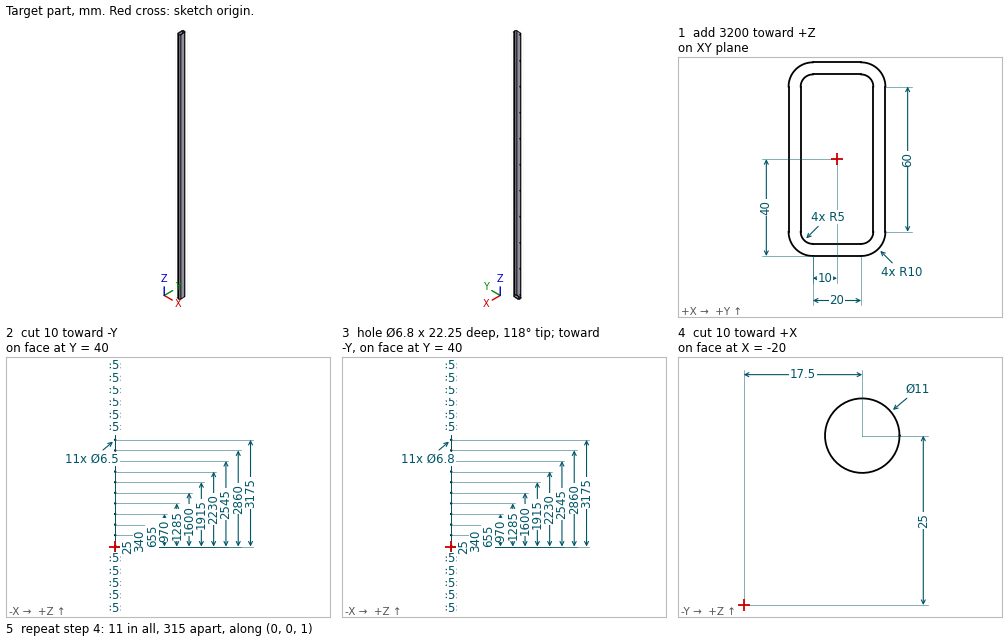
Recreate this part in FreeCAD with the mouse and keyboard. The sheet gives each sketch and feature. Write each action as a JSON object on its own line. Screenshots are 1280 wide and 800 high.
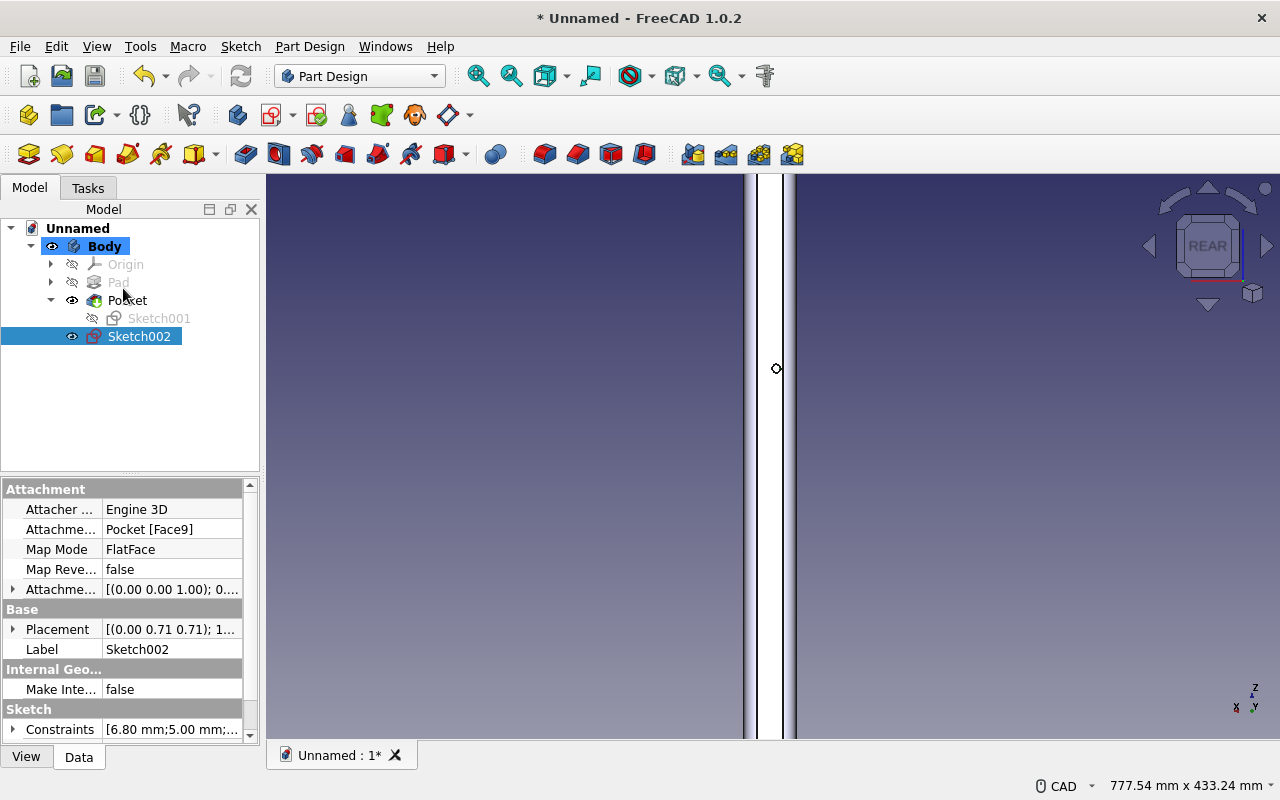
{"action": "left_click", "coordinate": [279, 154]}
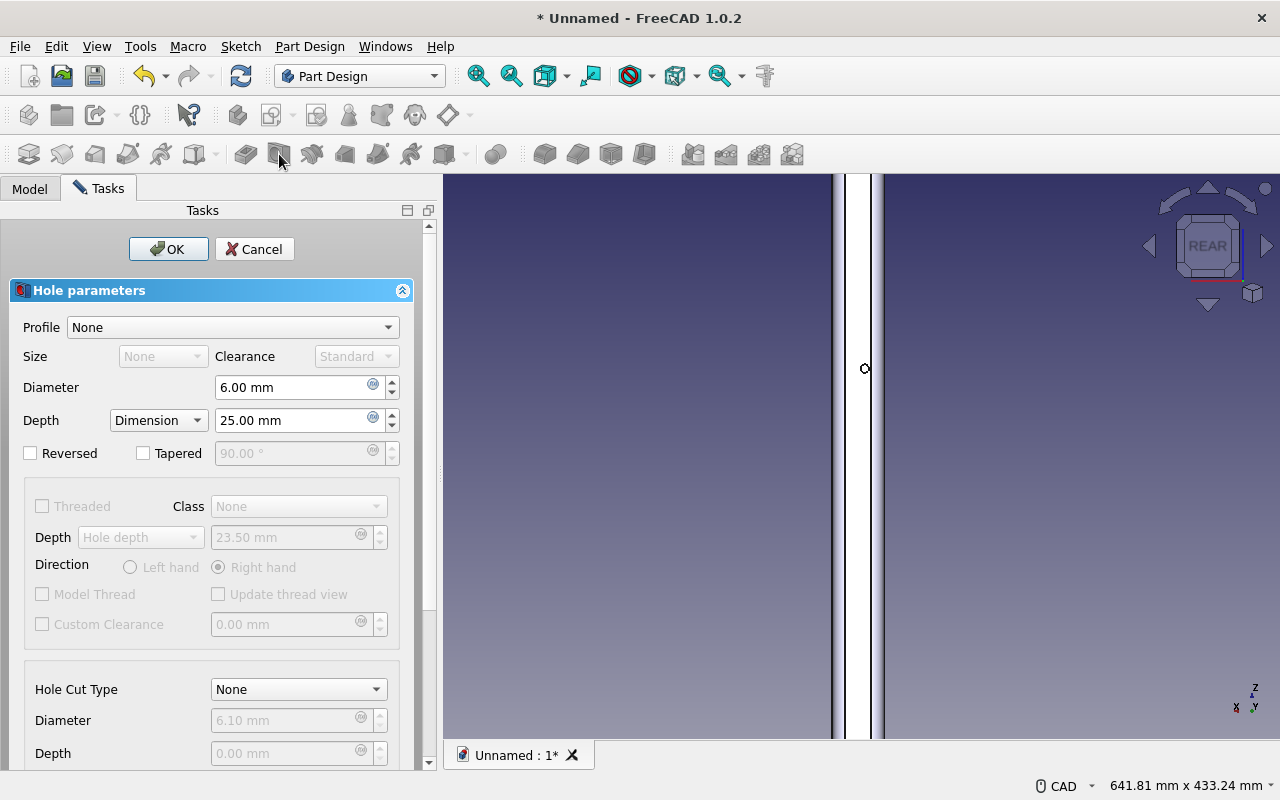
{"action": "triple_click", "coordinate": [300, 388]}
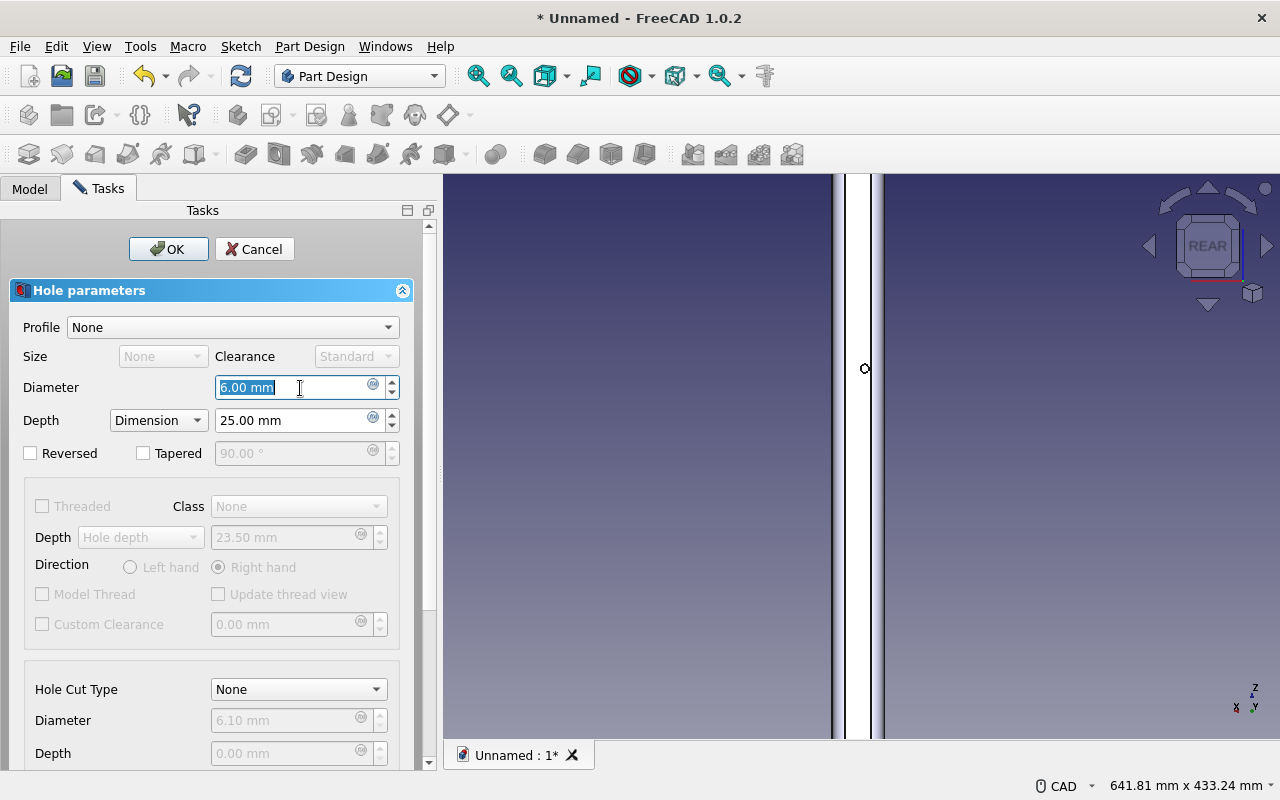
{"action": "type", "text": "6.8"}
{"action": "key", "text": "Tab"}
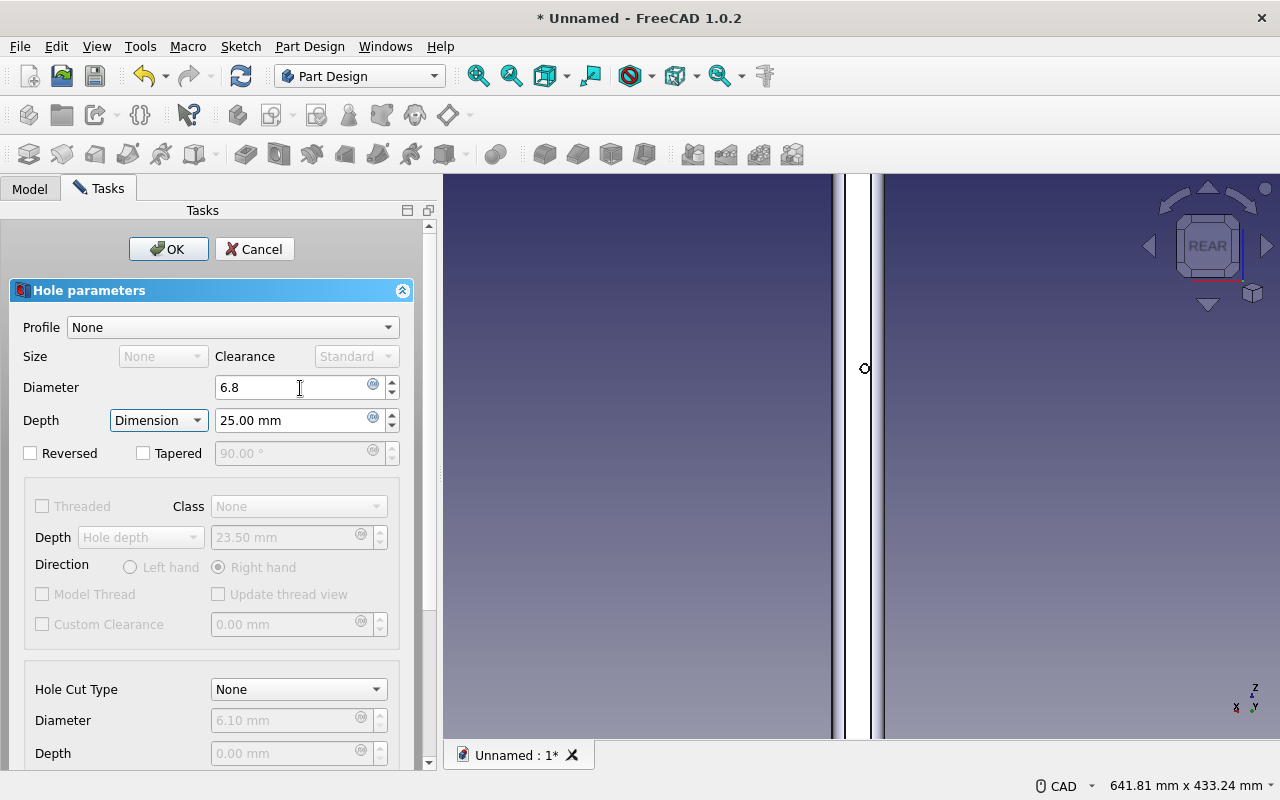
{"action": "triple_click", "coordinate": [300, 420]}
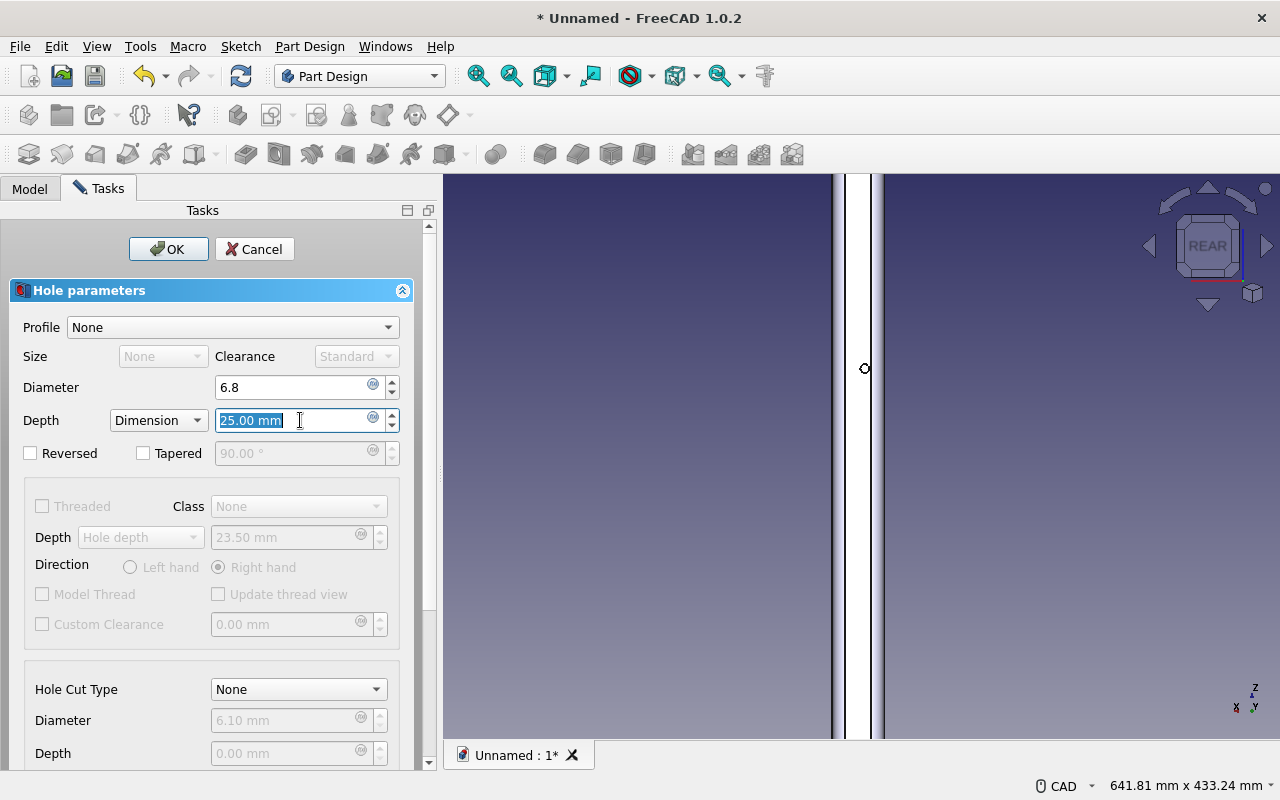
{"action": "type", "text": "22.25"}
{"action": "key", "text": "Tab"}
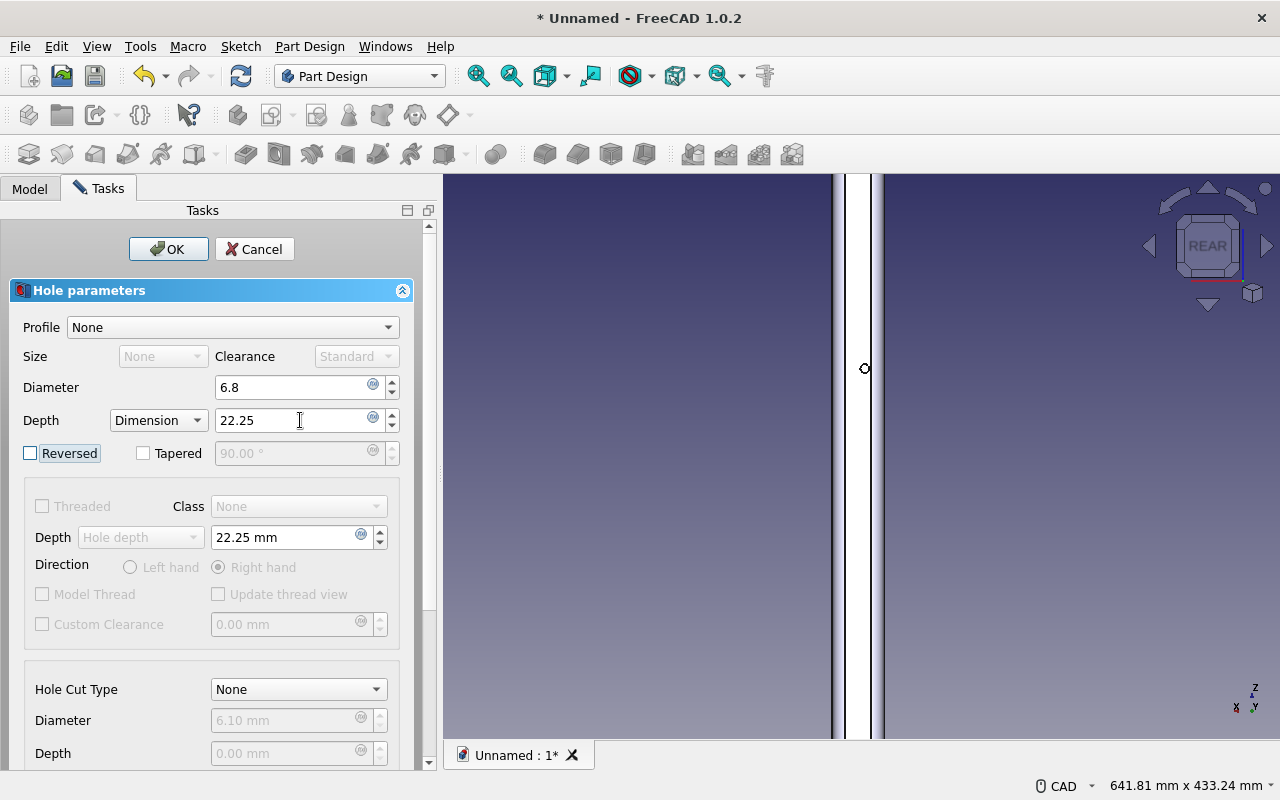
{"action": "left_click", "coordinate": [169, 249]}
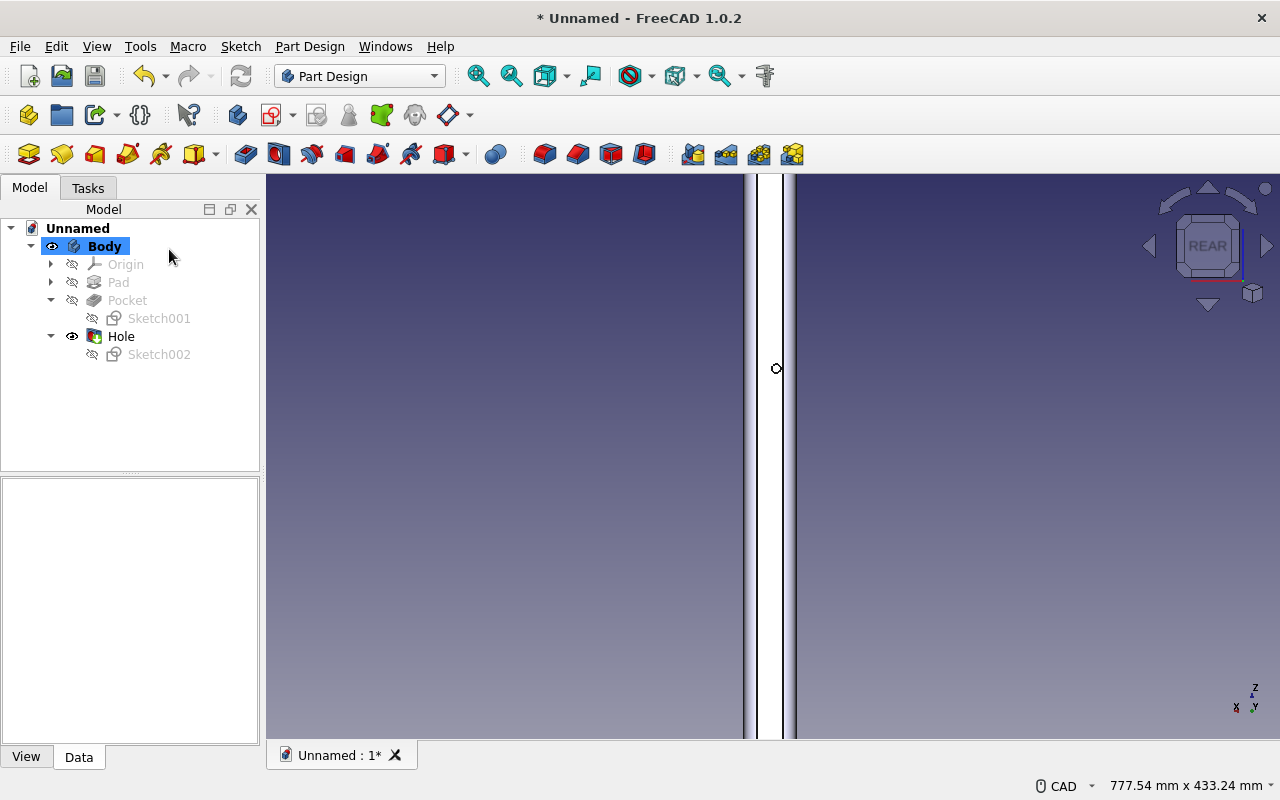
{"action": "left_click", "coordinate": [479, 76]}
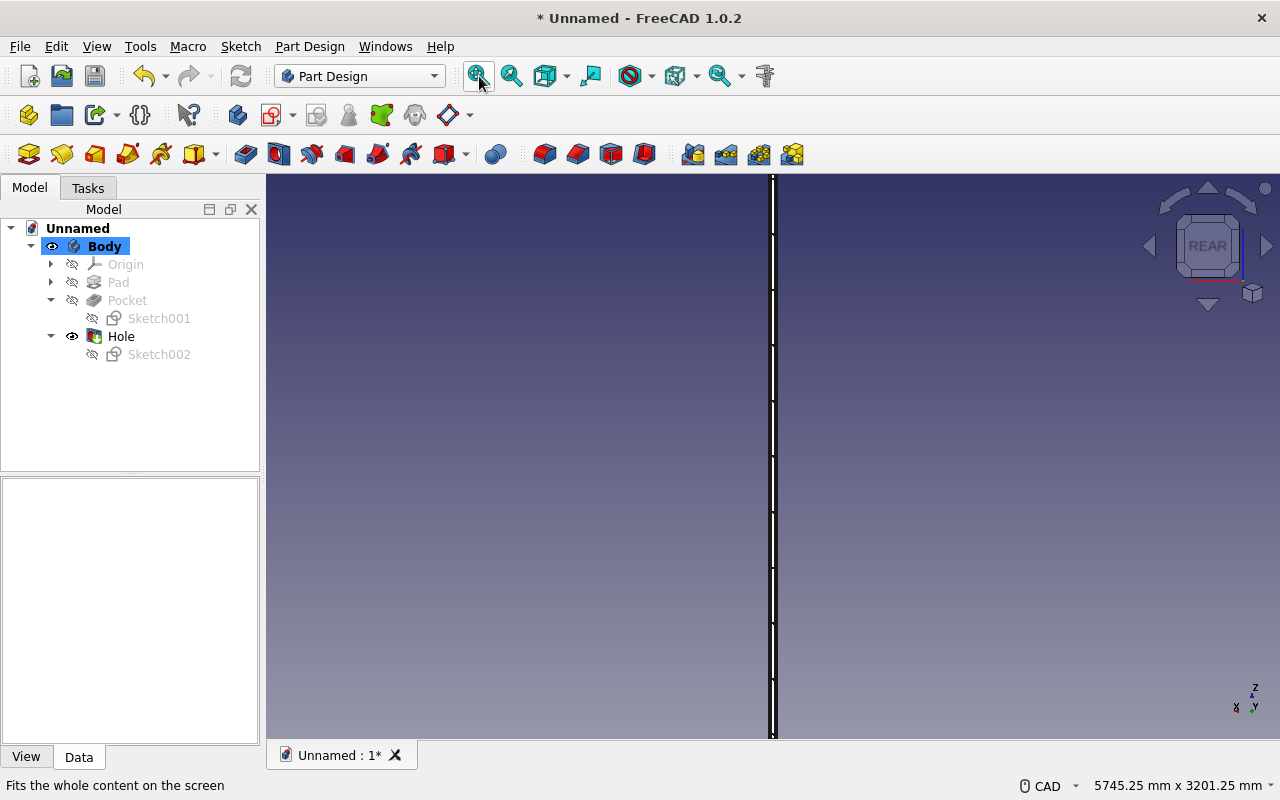
{"action": "key", "text": "6"}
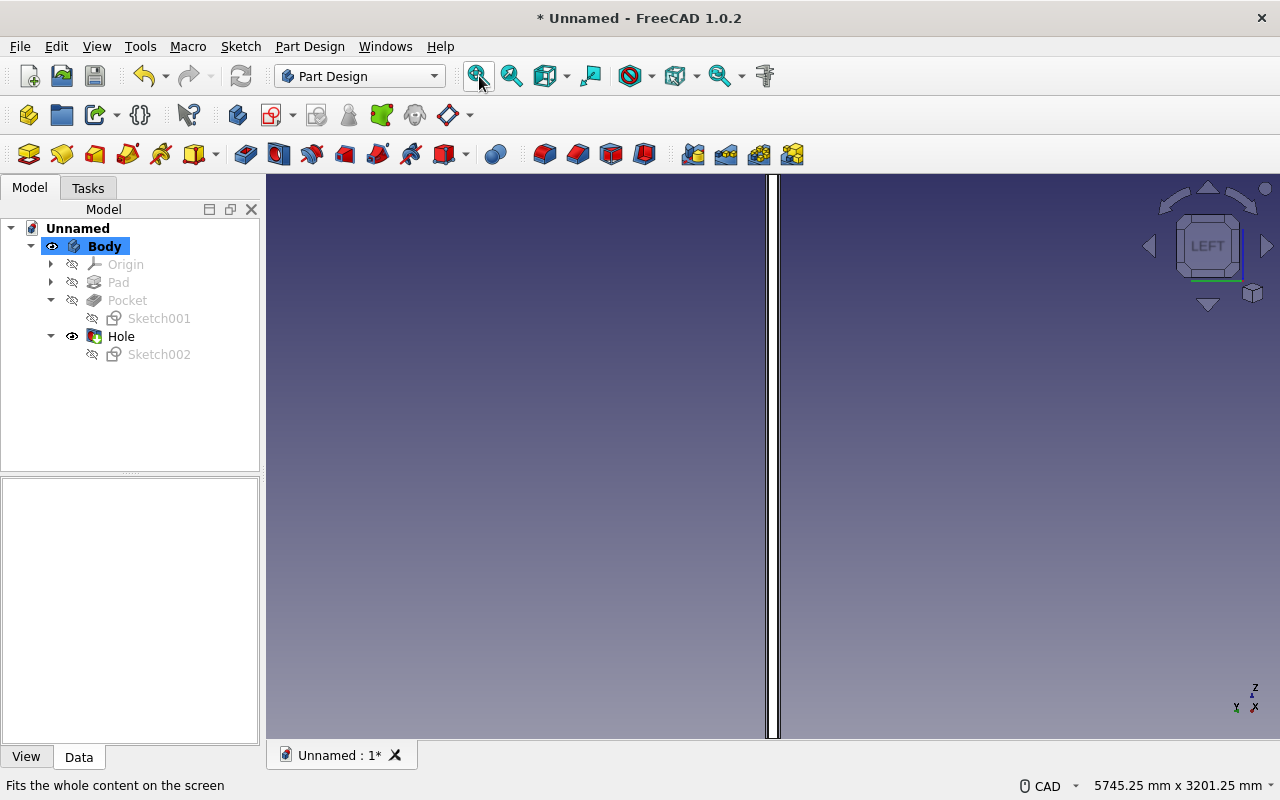
{"action": "left_click", "coordinate": [479, 76]}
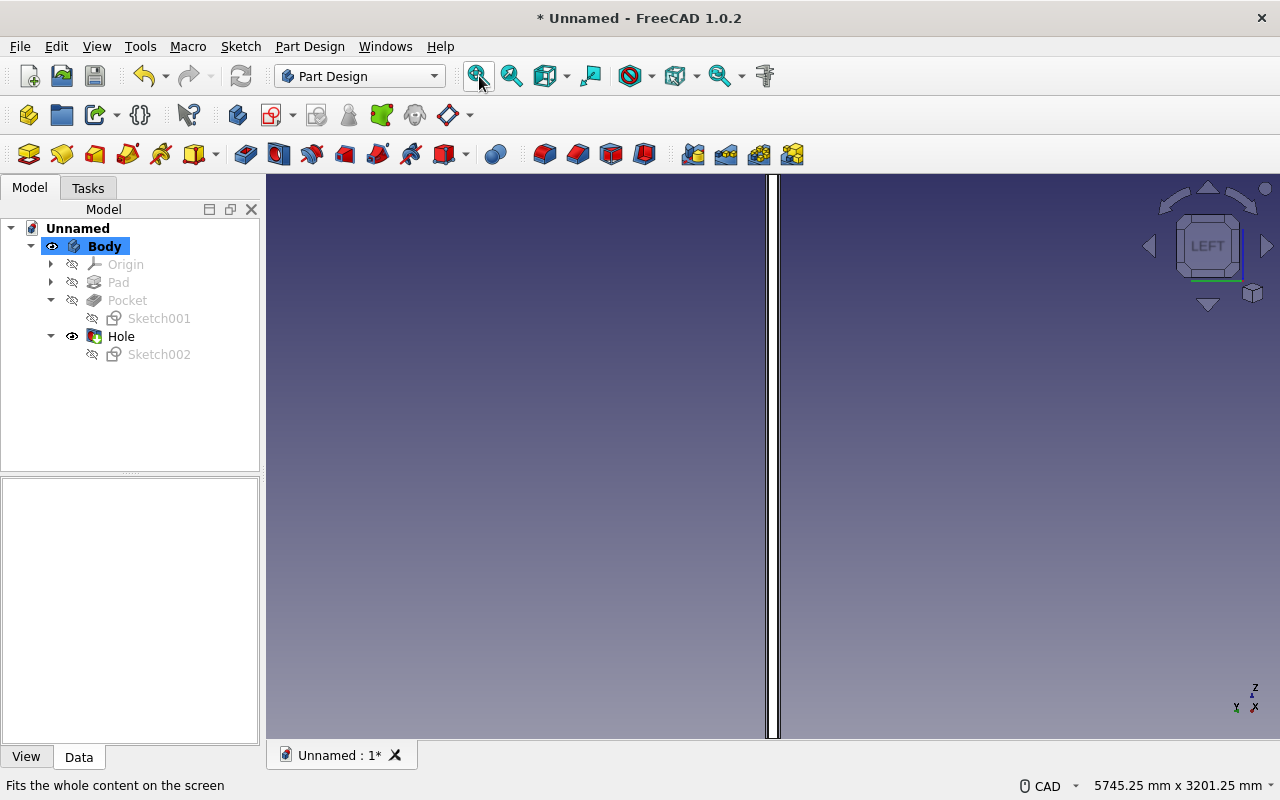
{"action": "scroll", "coordinate": [773, 213], "scroll_direction": "up", "scroll_amount": 5}